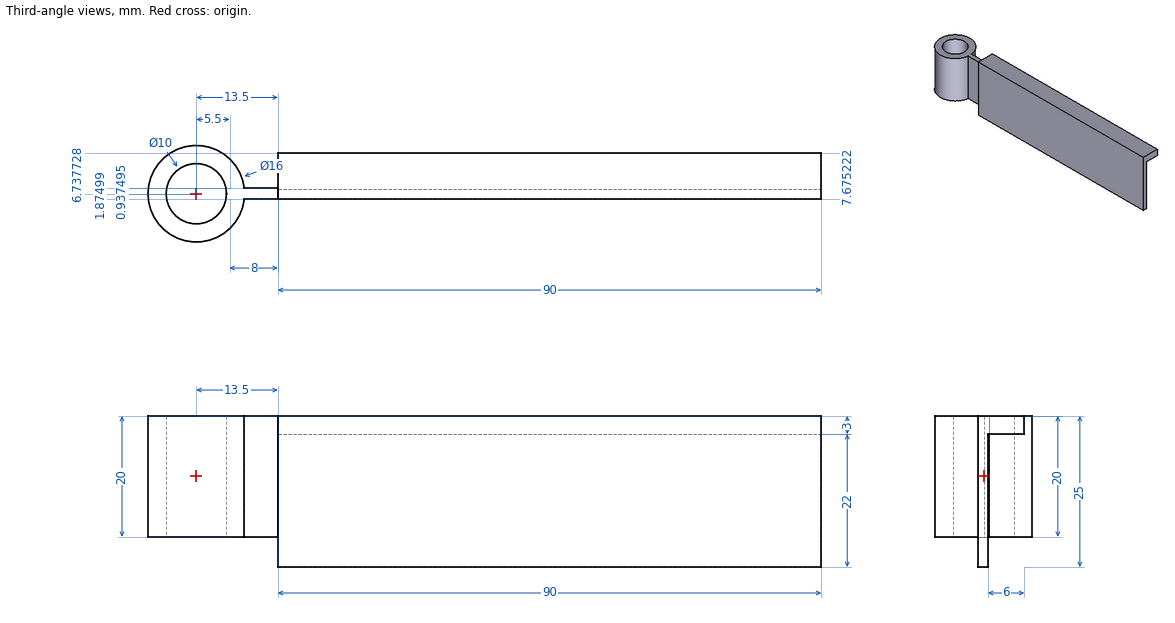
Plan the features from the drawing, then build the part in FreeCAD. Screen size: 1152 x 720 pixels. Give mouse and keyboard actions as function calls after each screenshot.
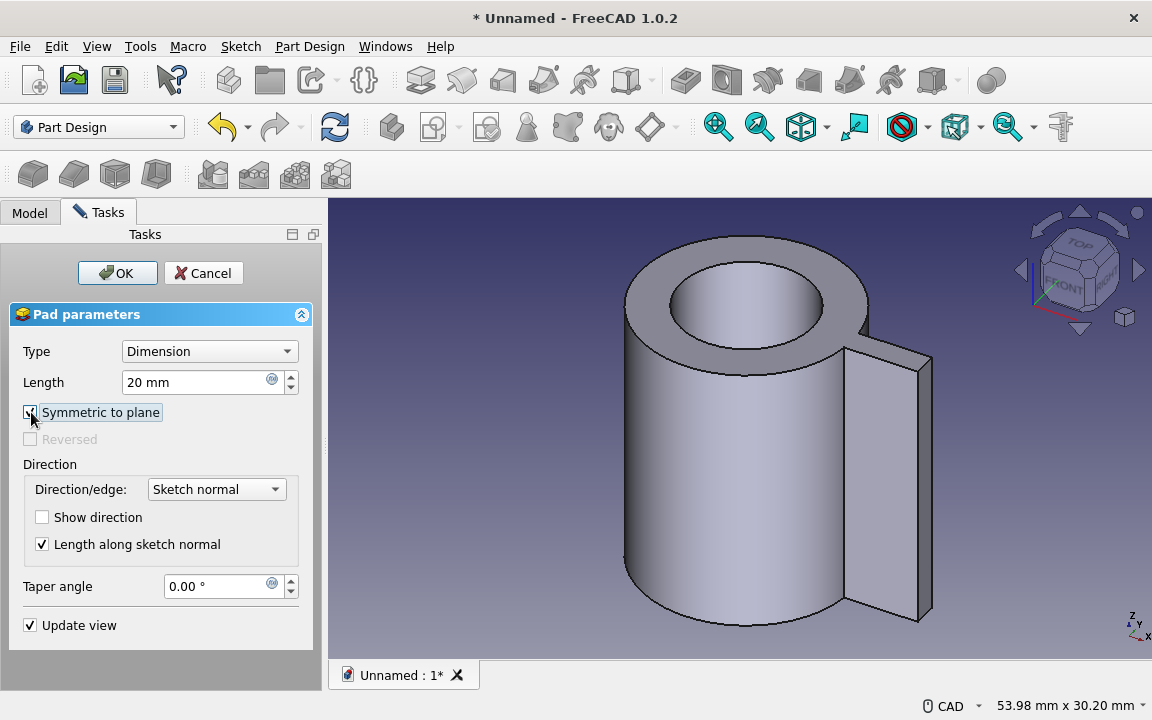
click(118, 273)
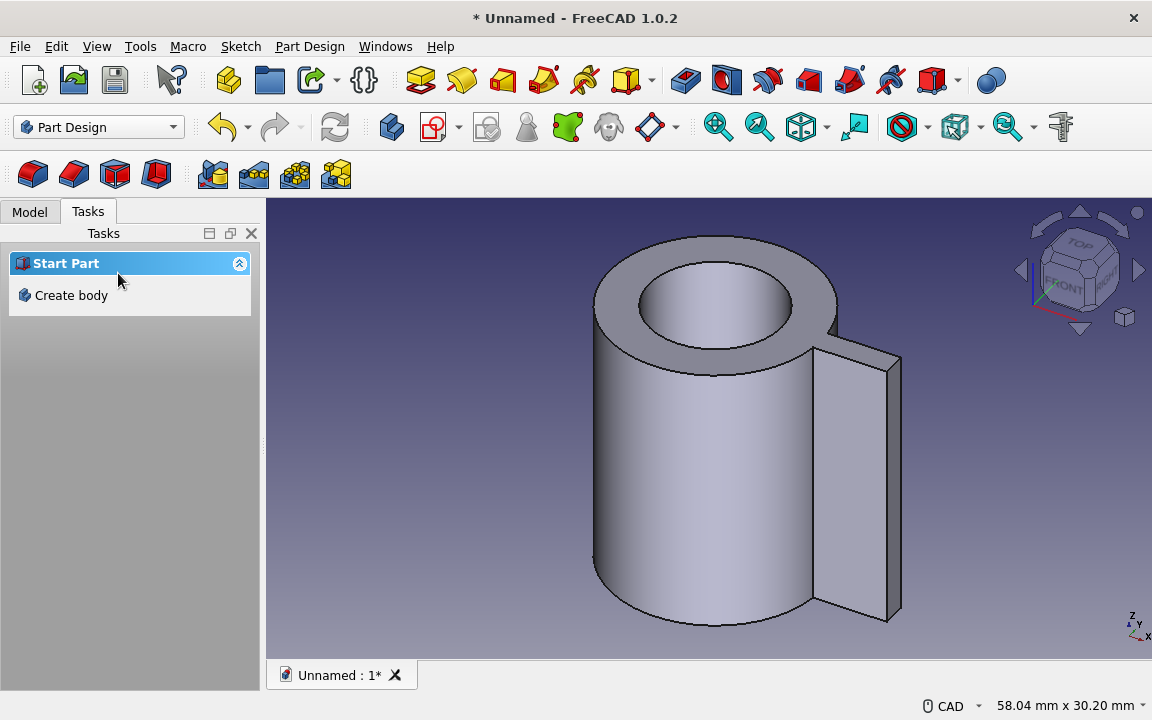
click(719, 128)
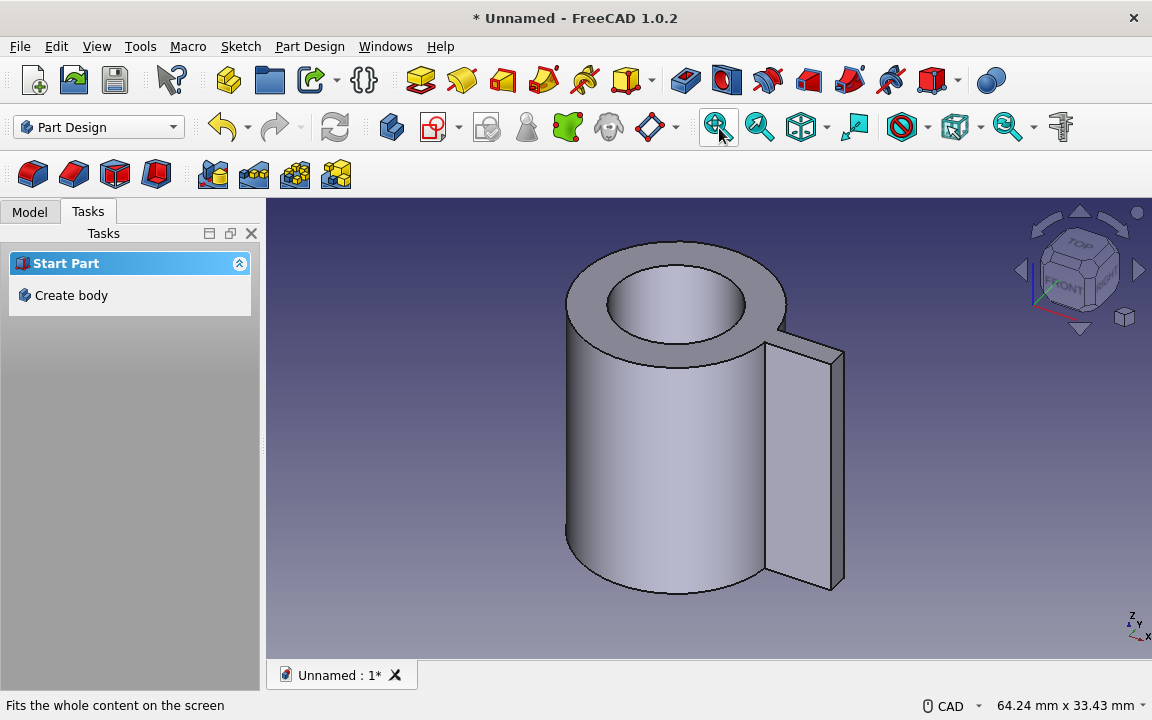
click(392, 128)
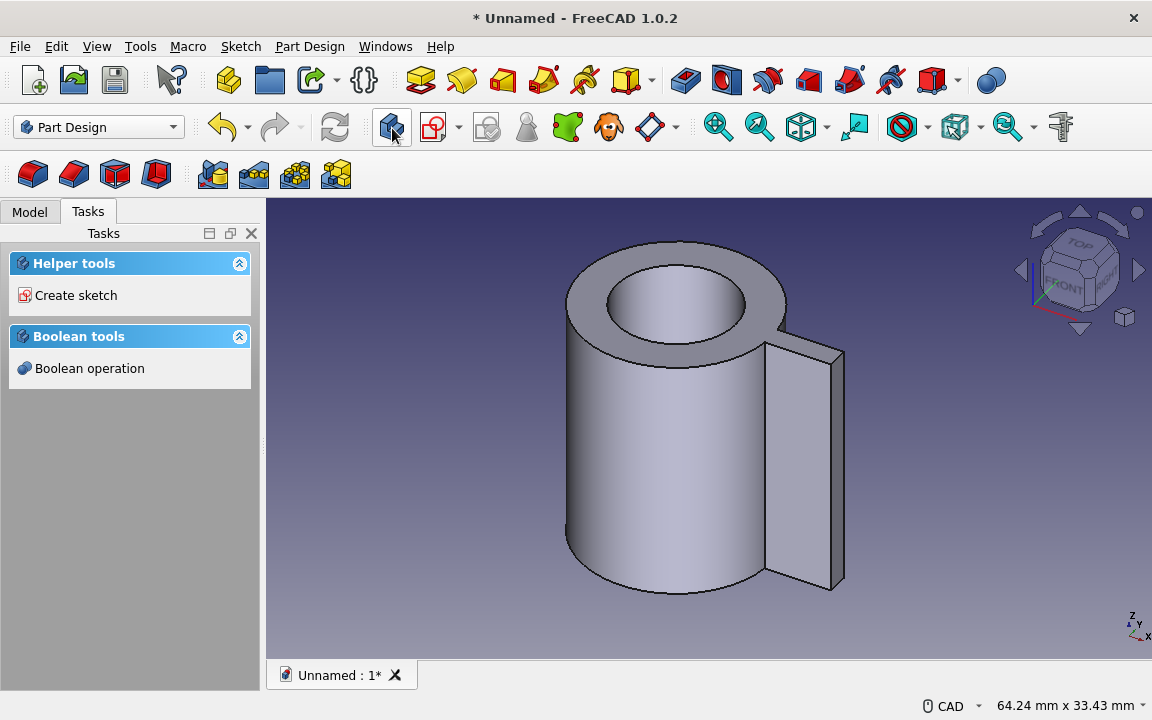
click(30, 212)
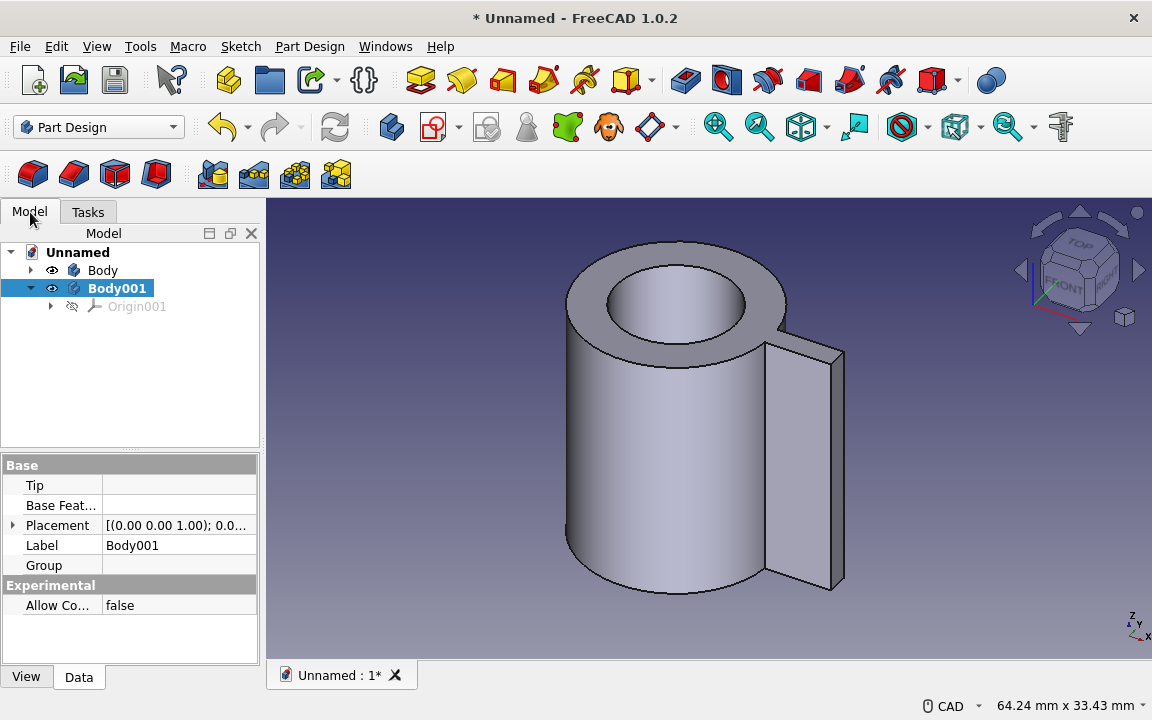
click(51, 306)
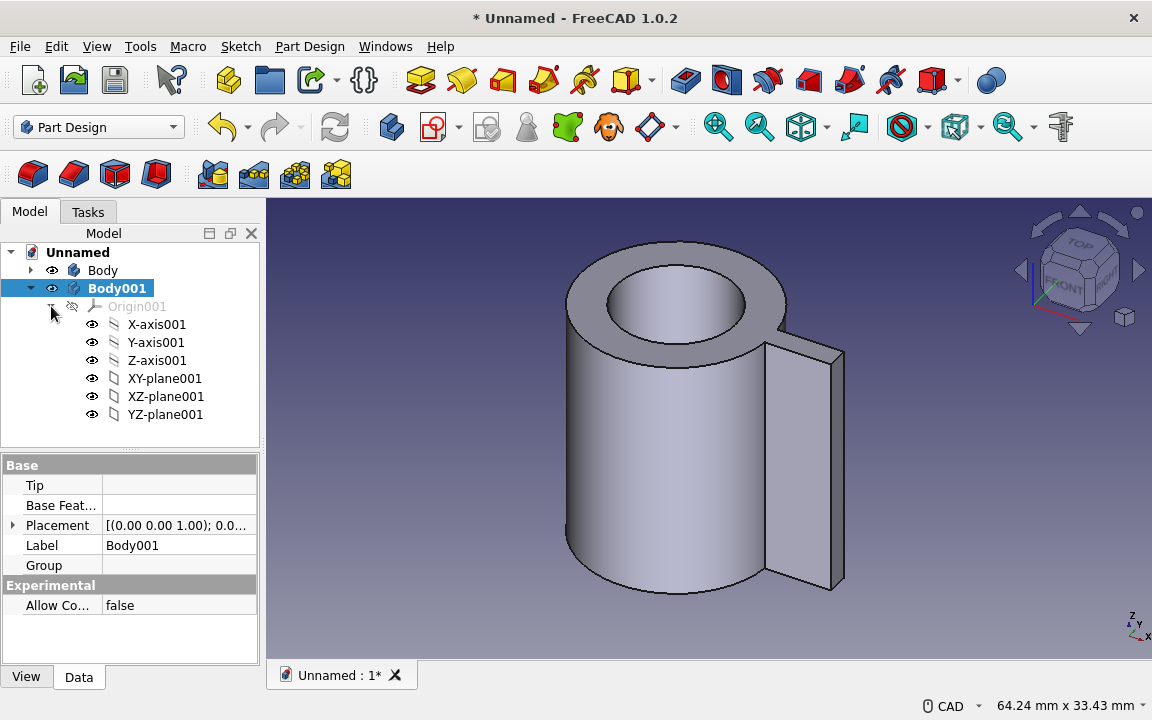
click(137, 378)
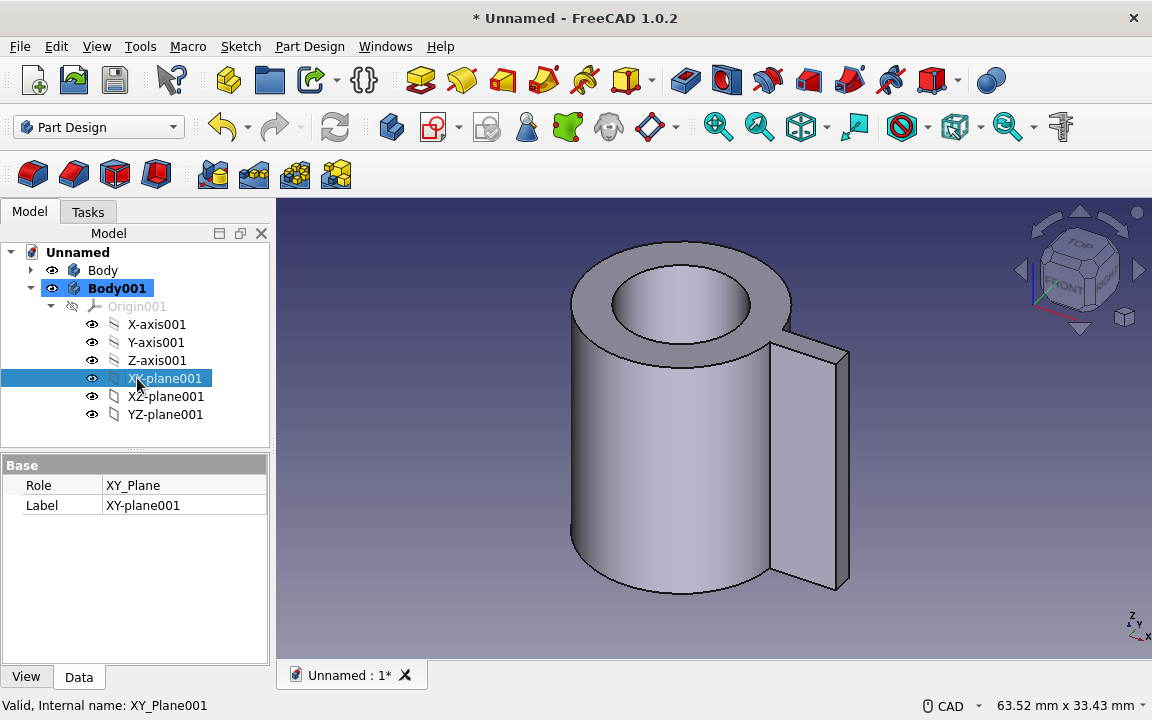
click(650, 128)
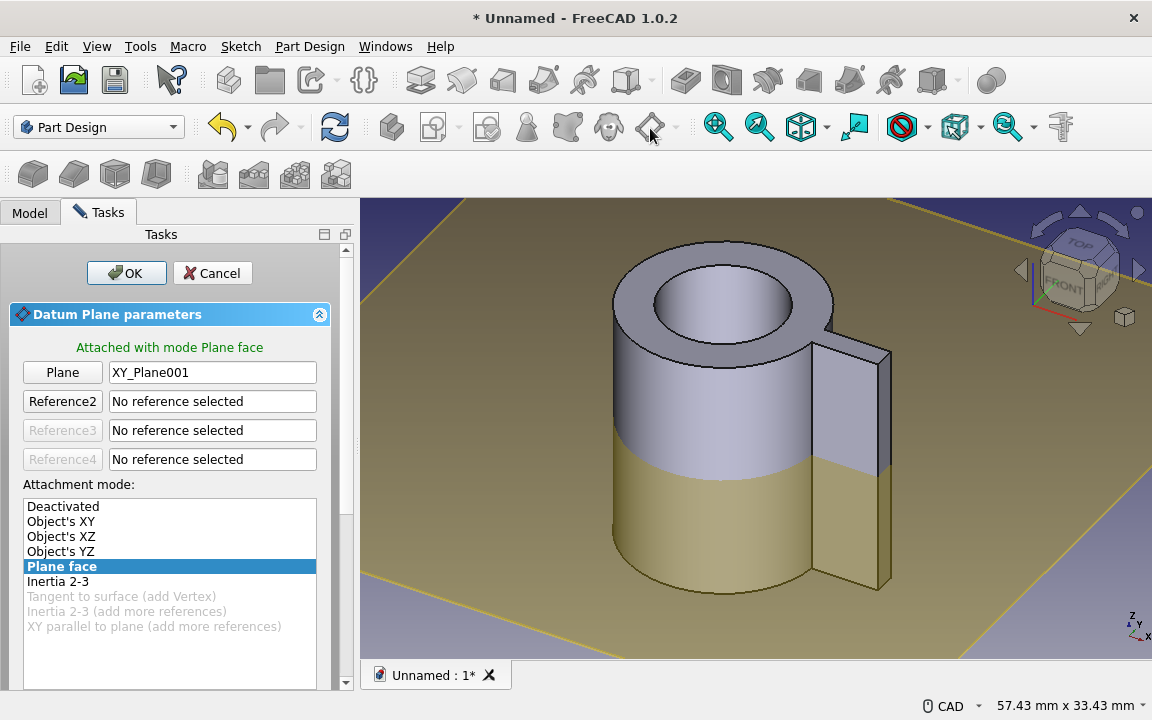
scroll(346, 467, down, 4)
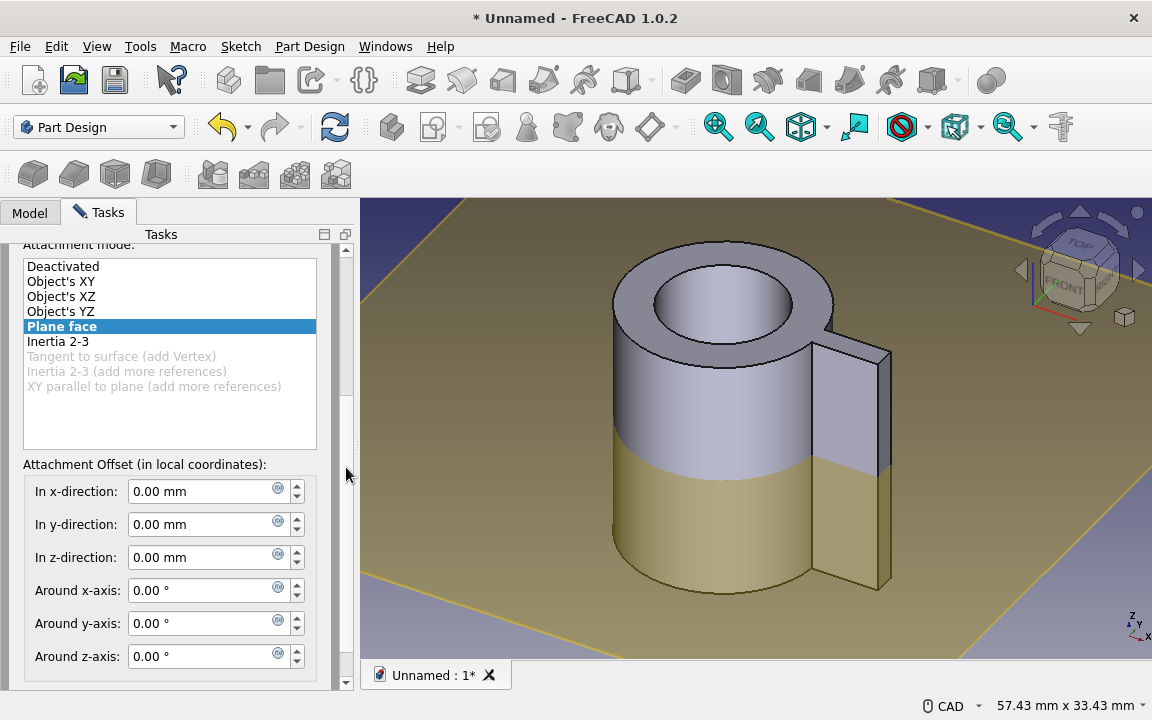
triple_click(210, 558)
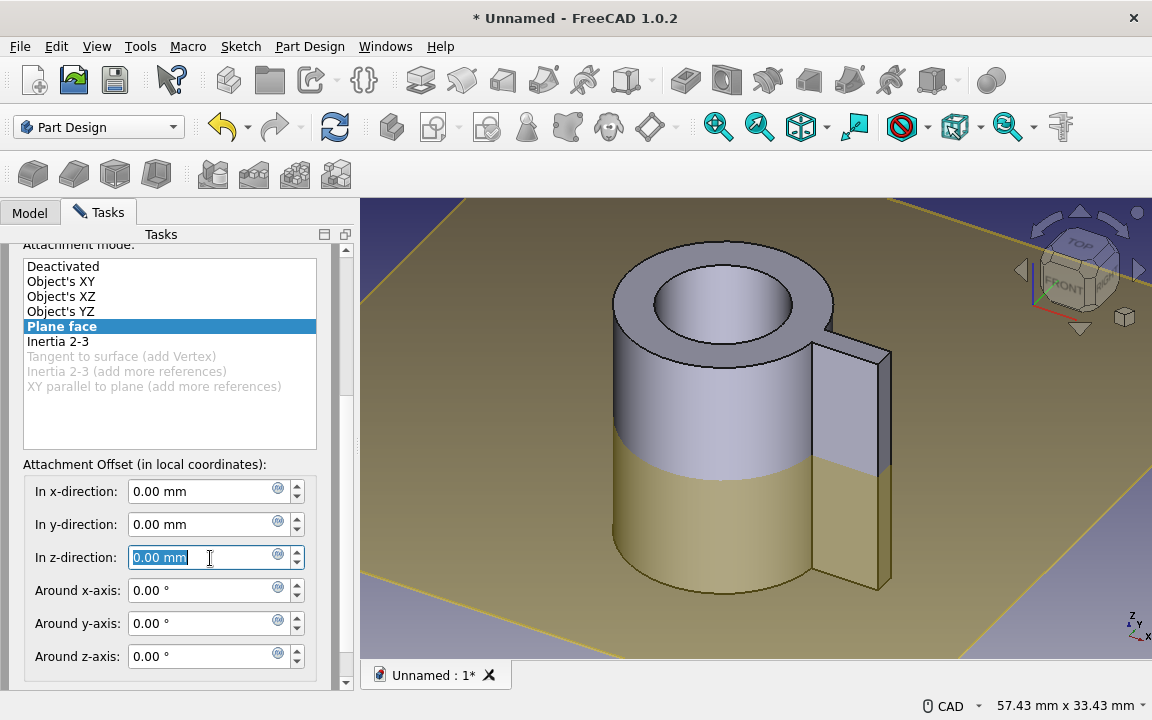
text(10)
key(Tab)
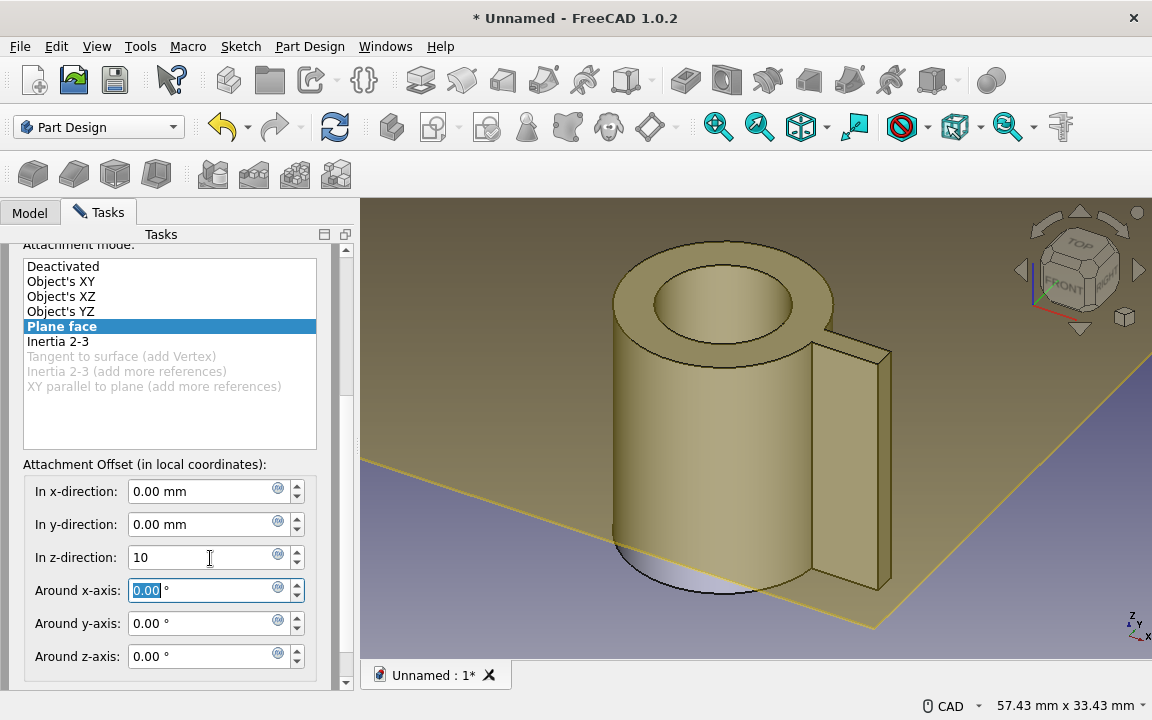
scroll(346, 467, up, 5)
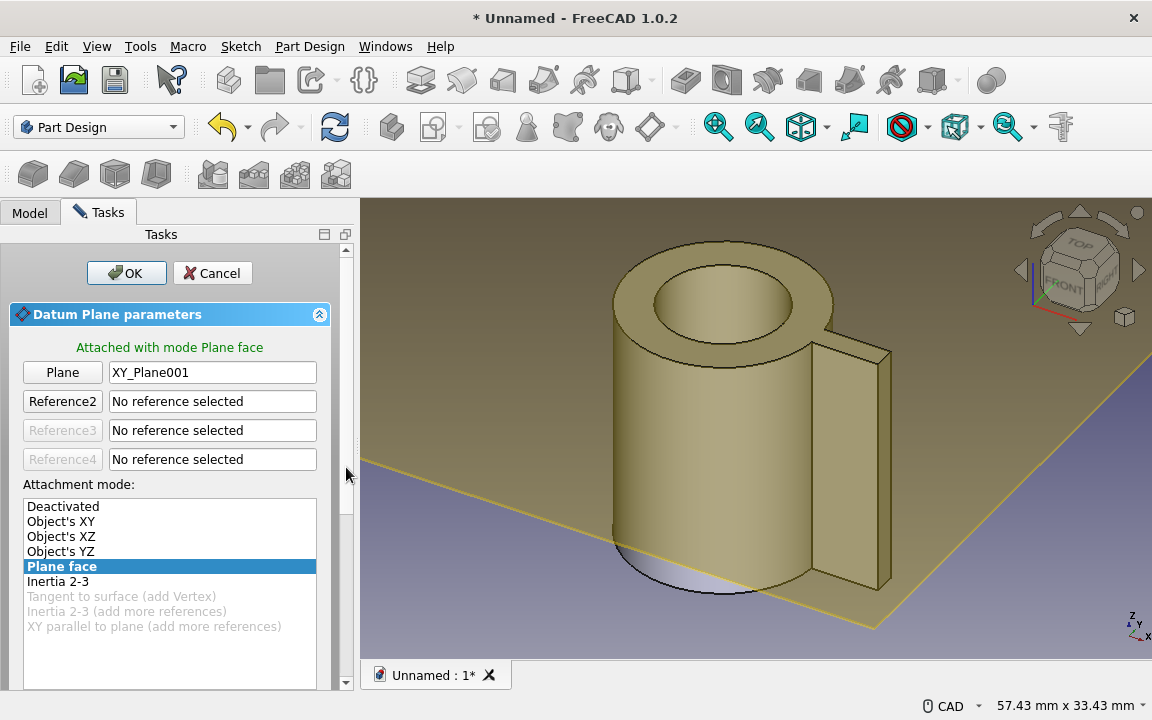
click(127, 273)